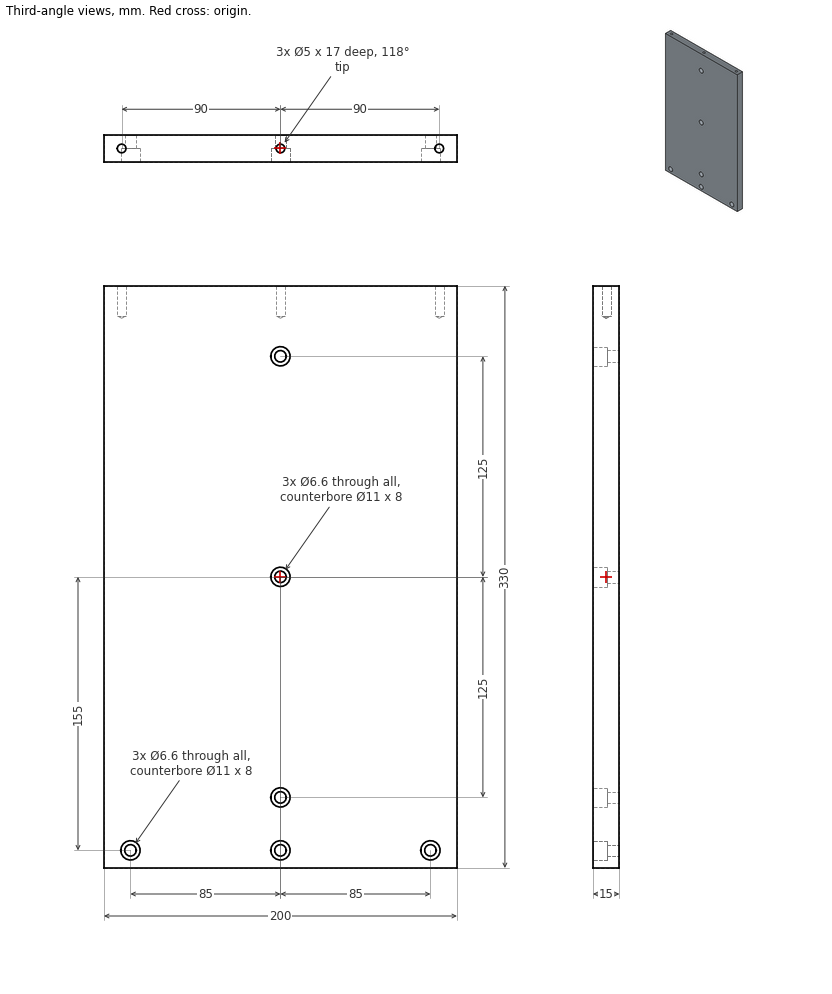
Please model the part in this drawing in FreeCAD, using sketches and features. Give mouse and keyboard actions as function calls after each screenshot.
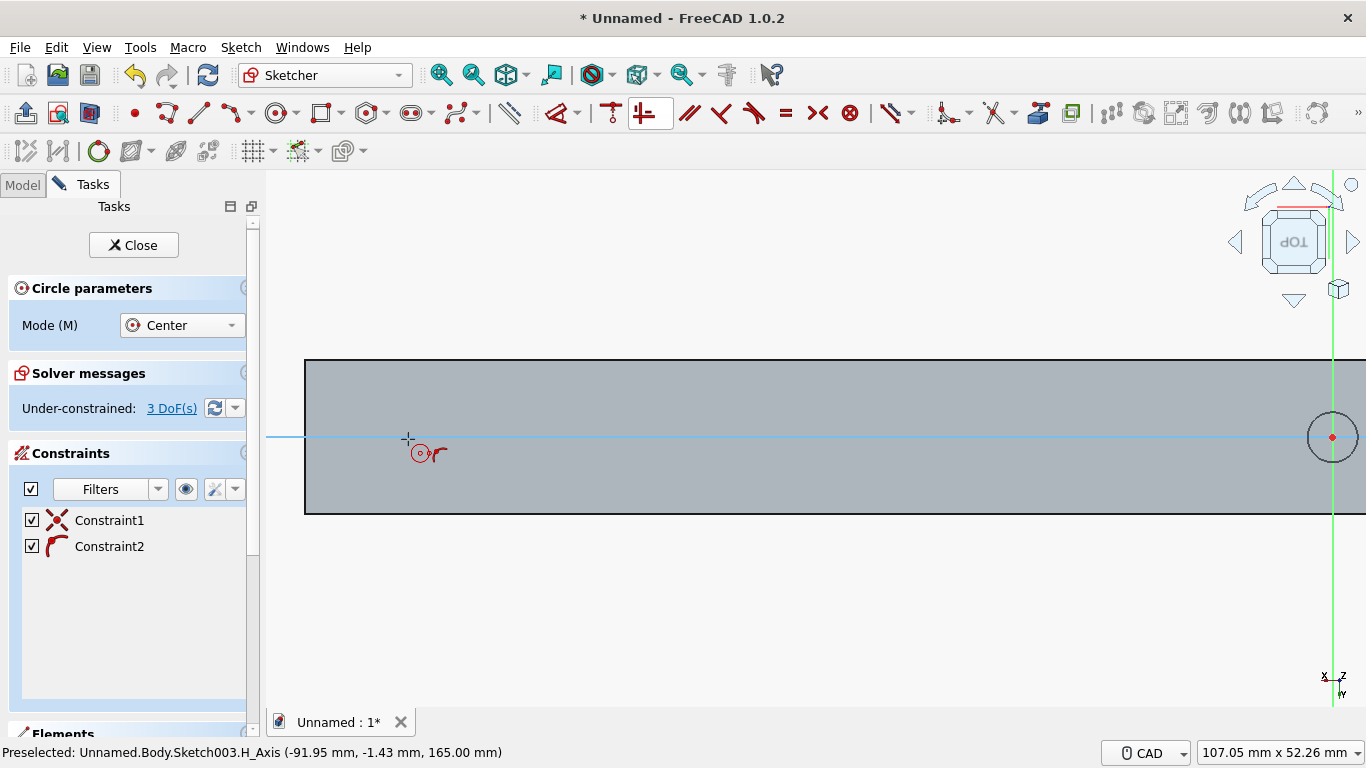
click(408, 437)
click(426, 419)
key(Escape)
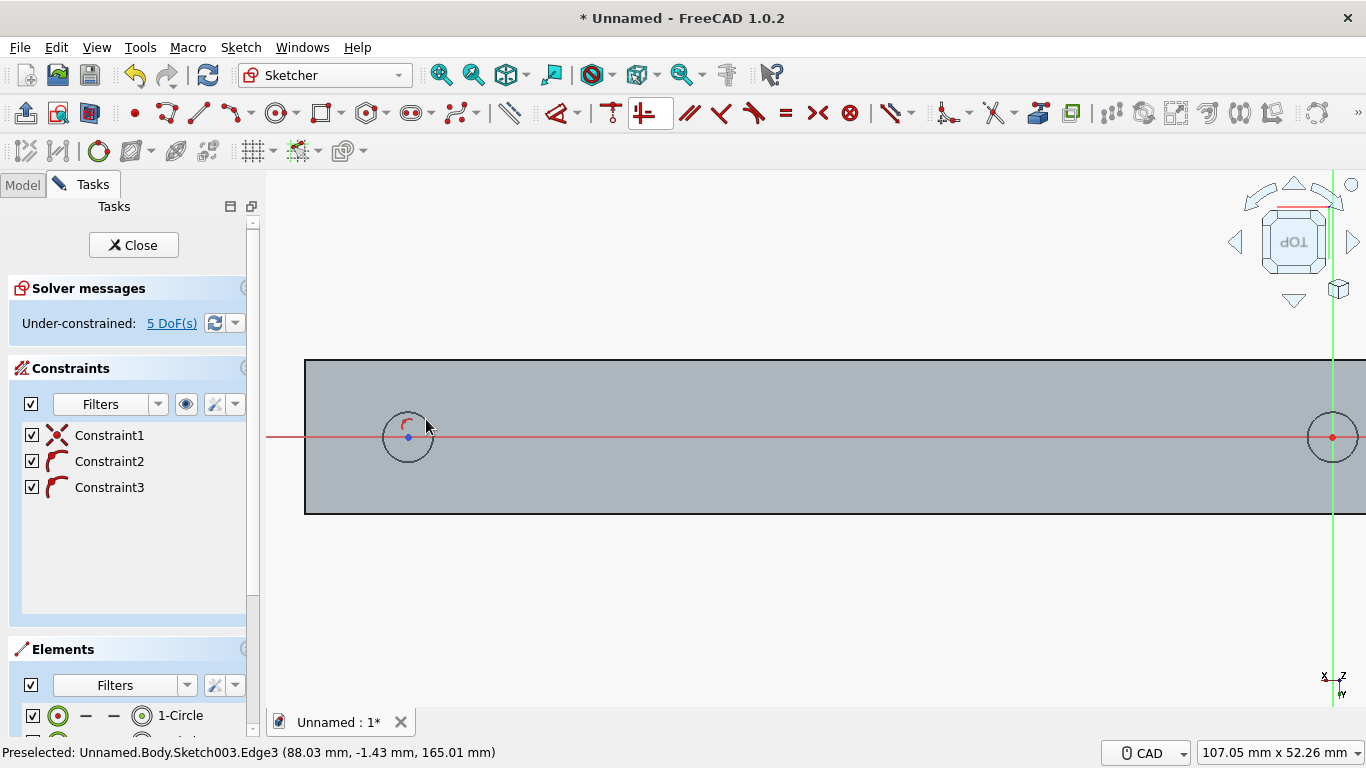
scroll(407, 439, down, 5)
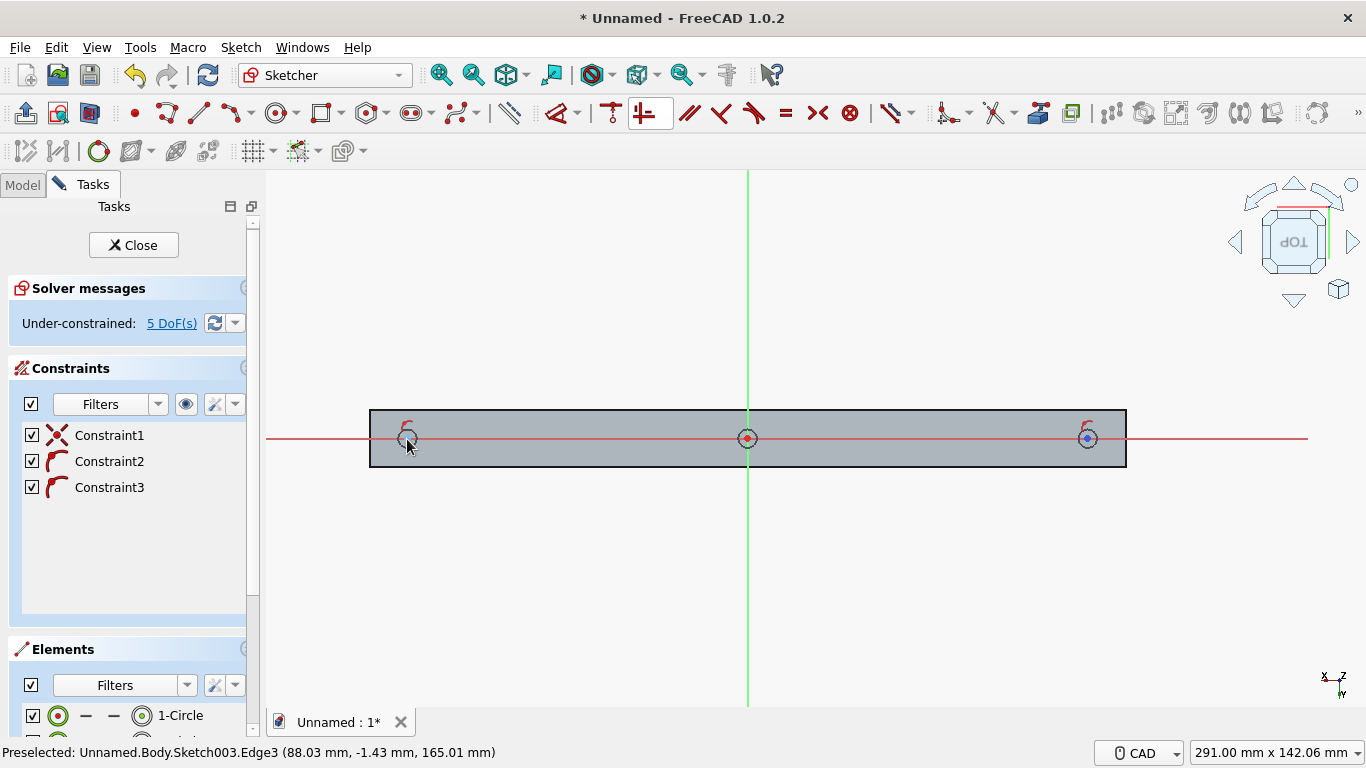
scroll(754, 432, up, 4)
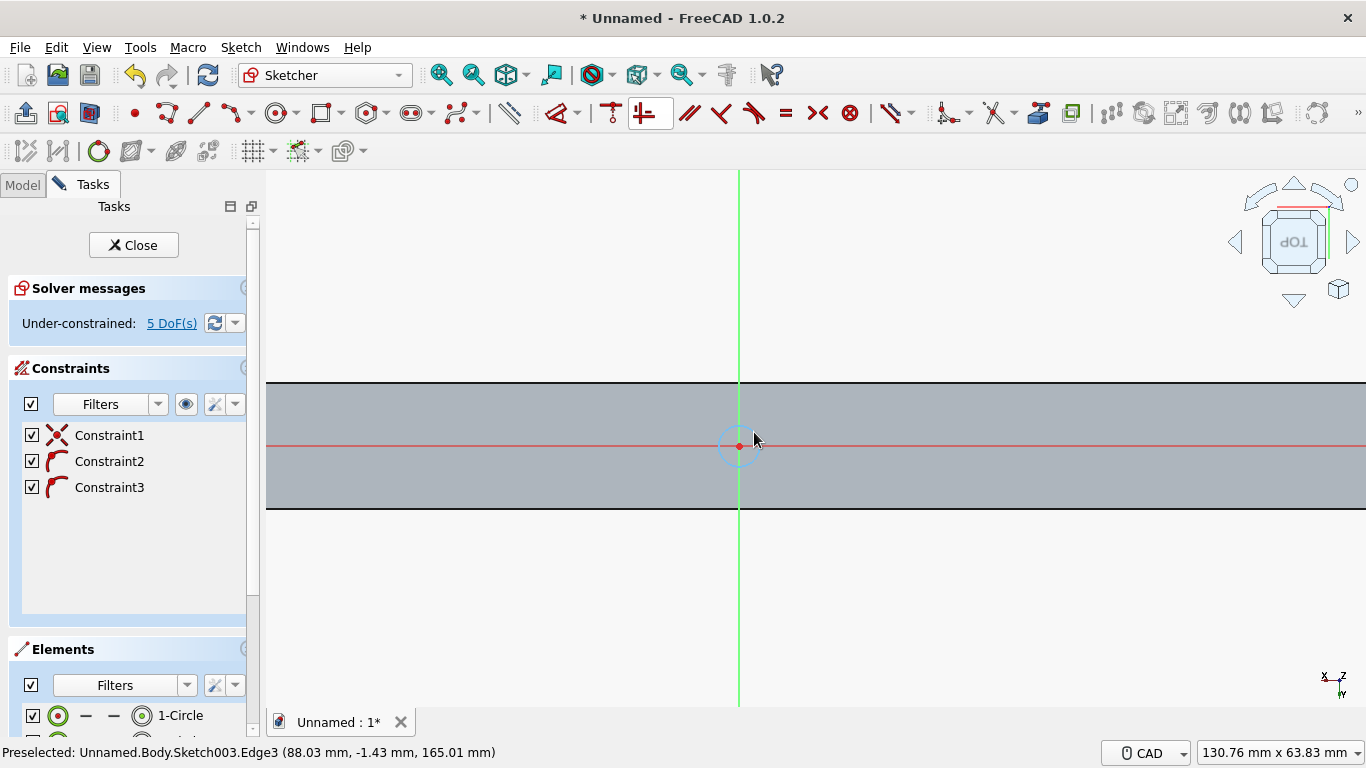
click(754, 432)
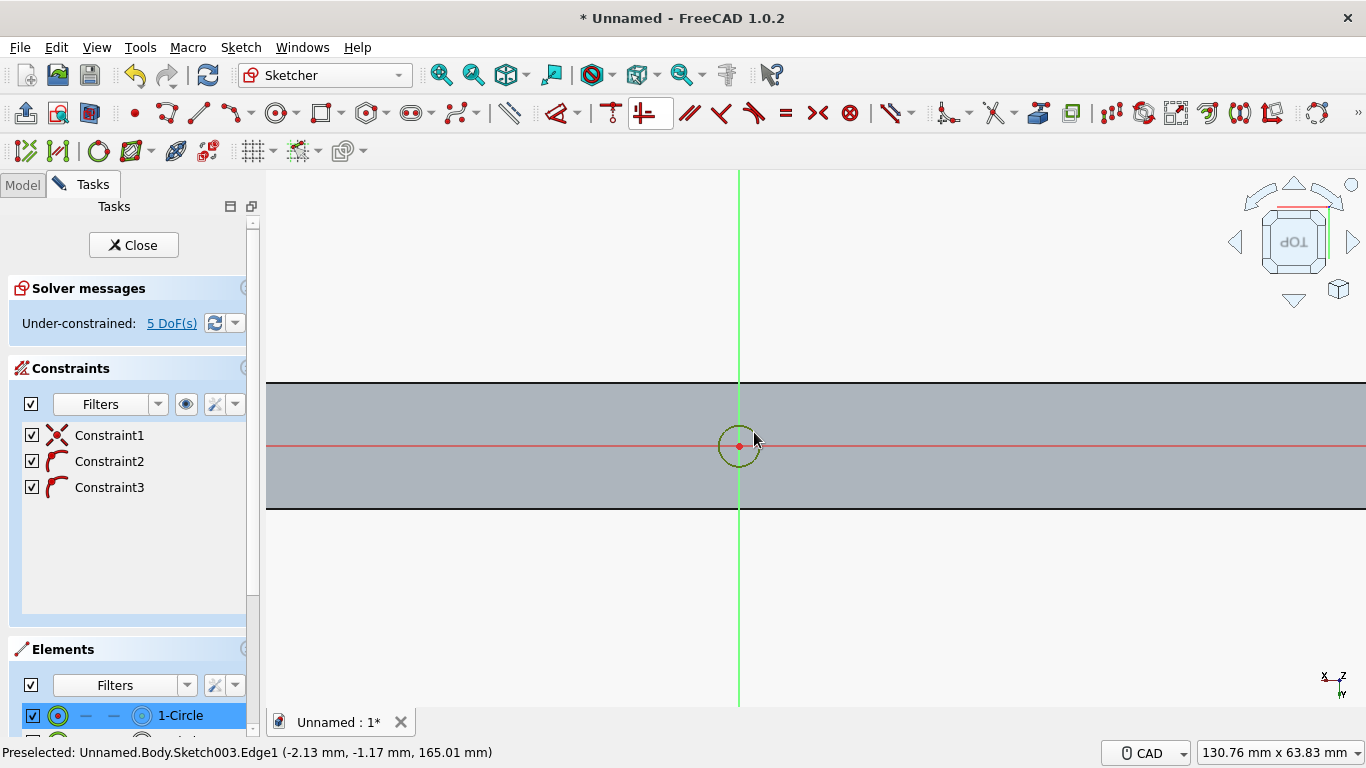
scroll(754, 432, down, 4)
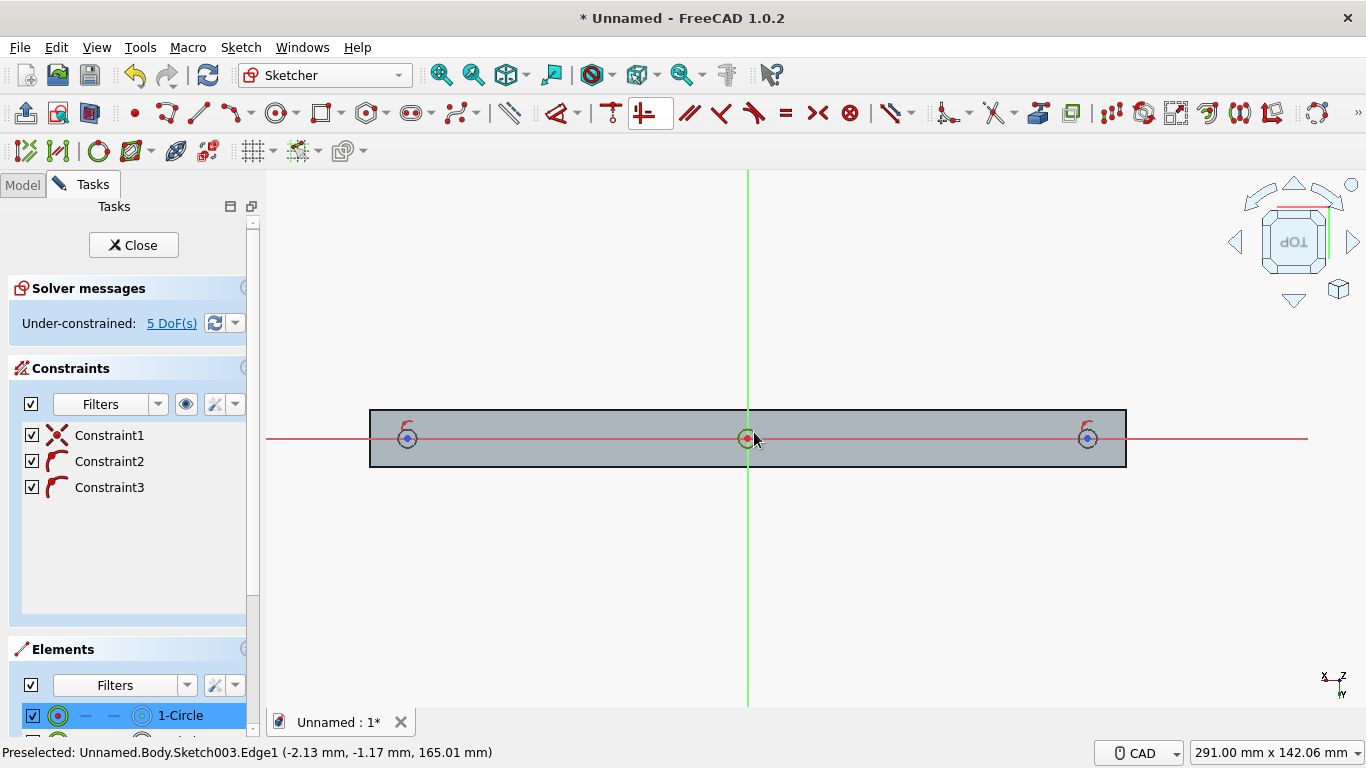
scroll(1094, 432, up, 4)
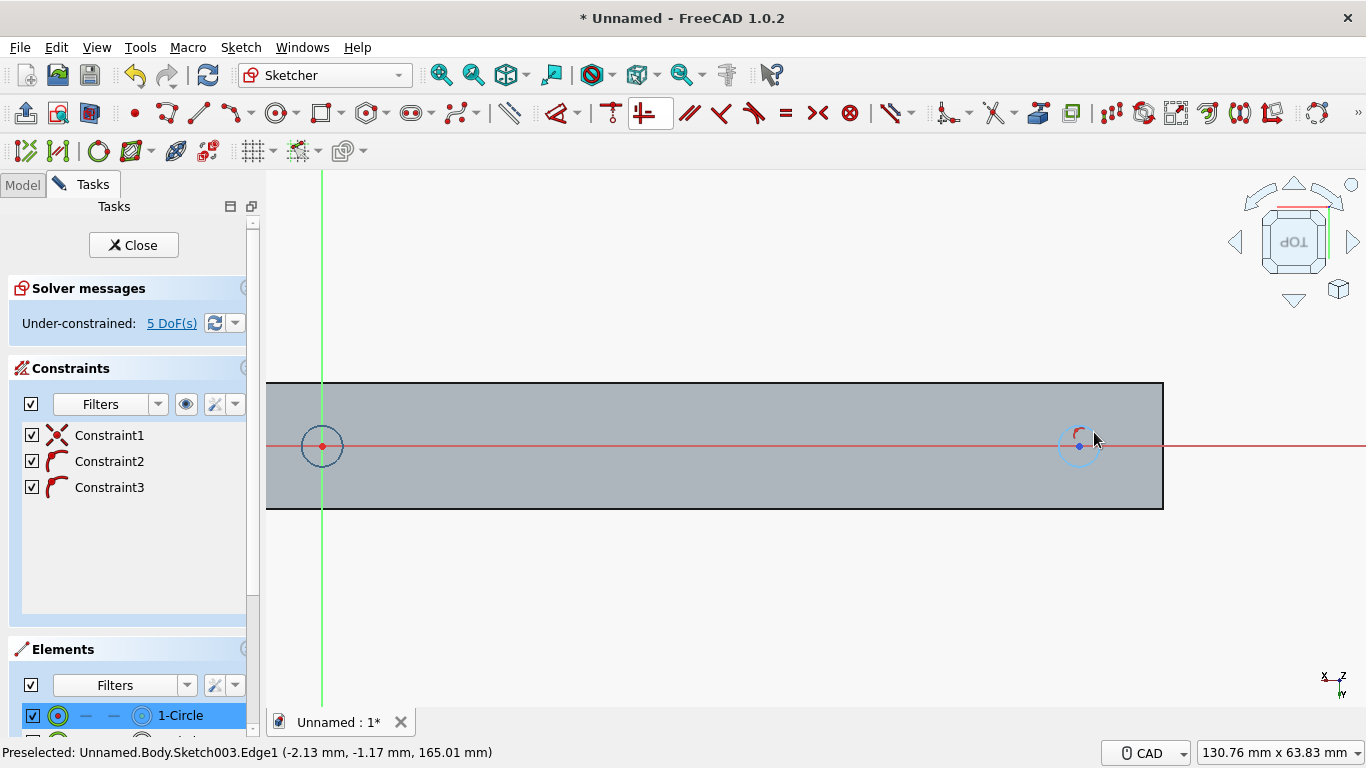
click(1094, 432)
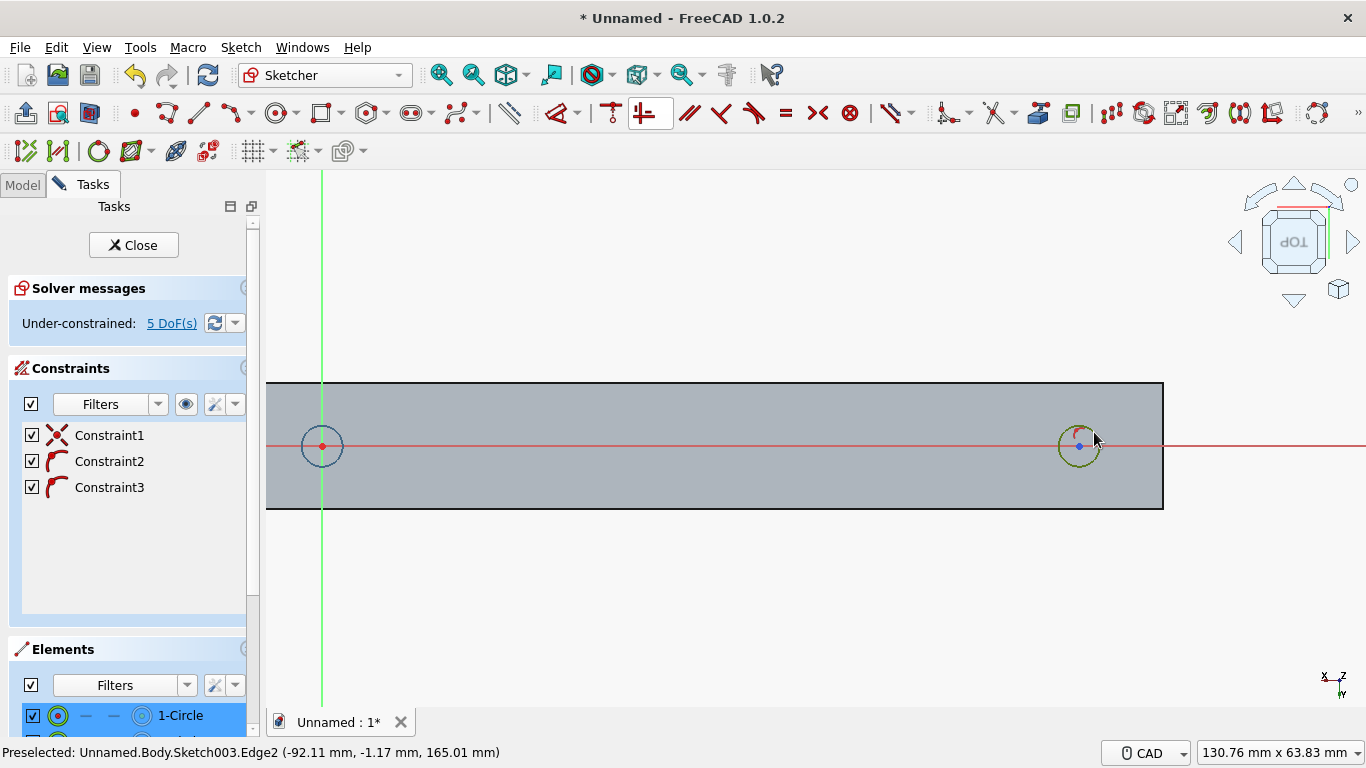
scroll(1095, 432, down, 4)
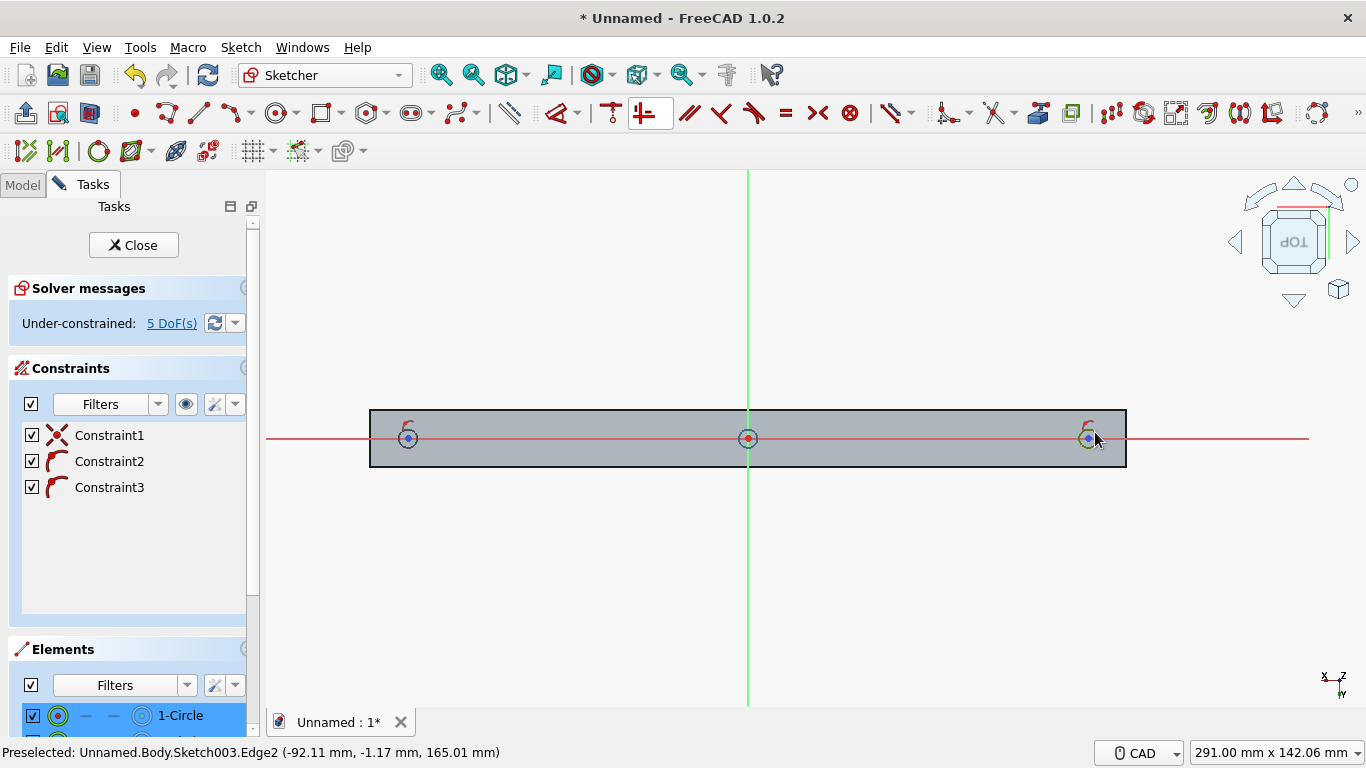
scroll(414, 432, up, 4)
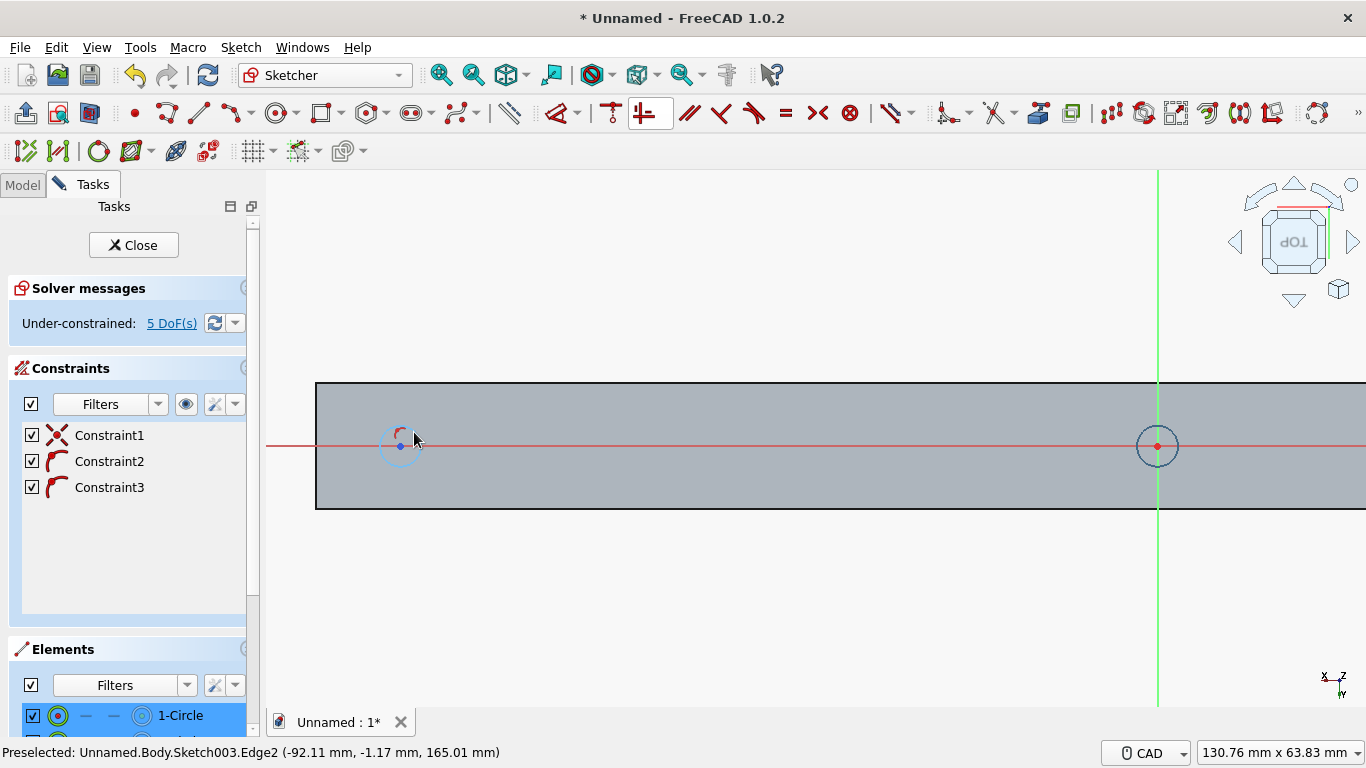
click(415, 432)